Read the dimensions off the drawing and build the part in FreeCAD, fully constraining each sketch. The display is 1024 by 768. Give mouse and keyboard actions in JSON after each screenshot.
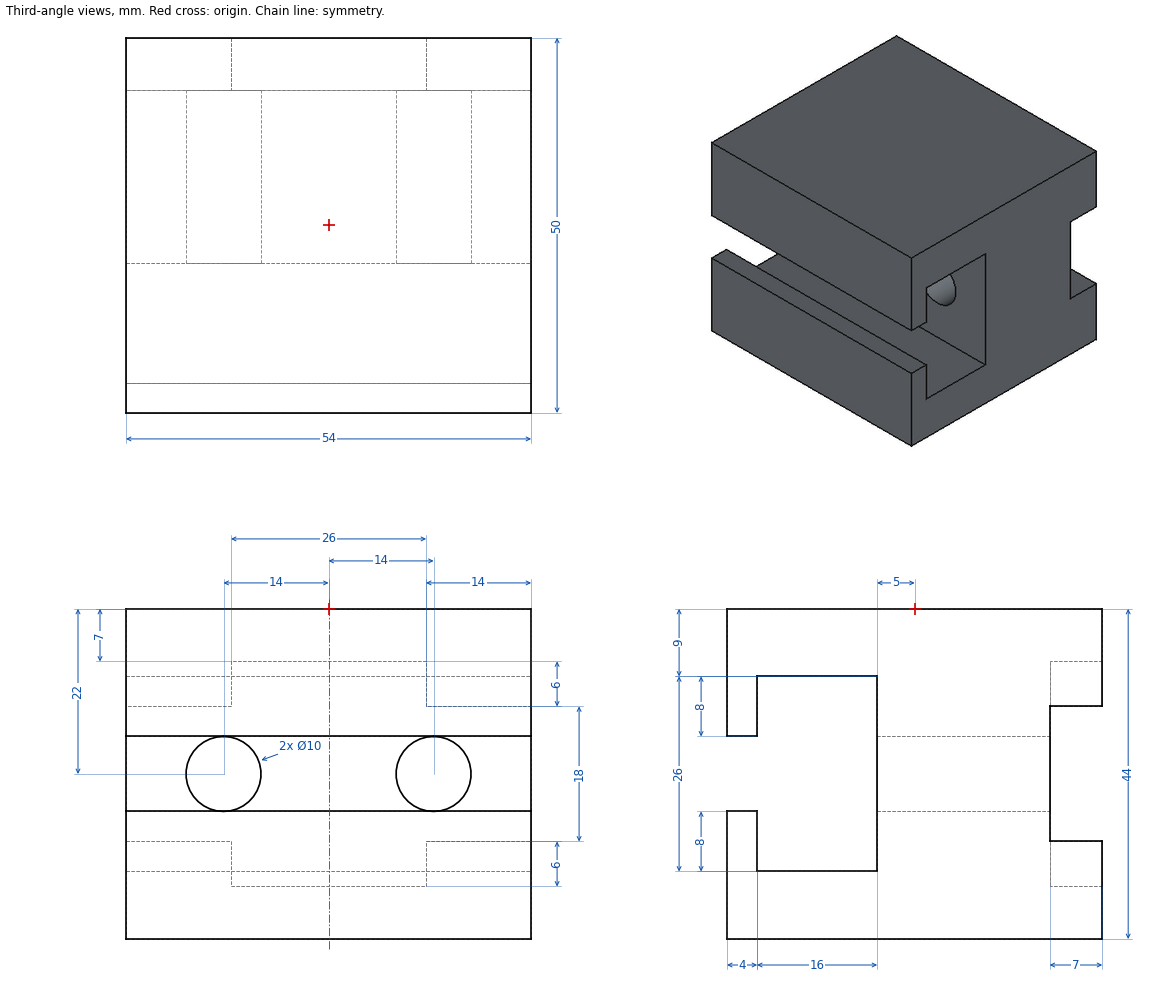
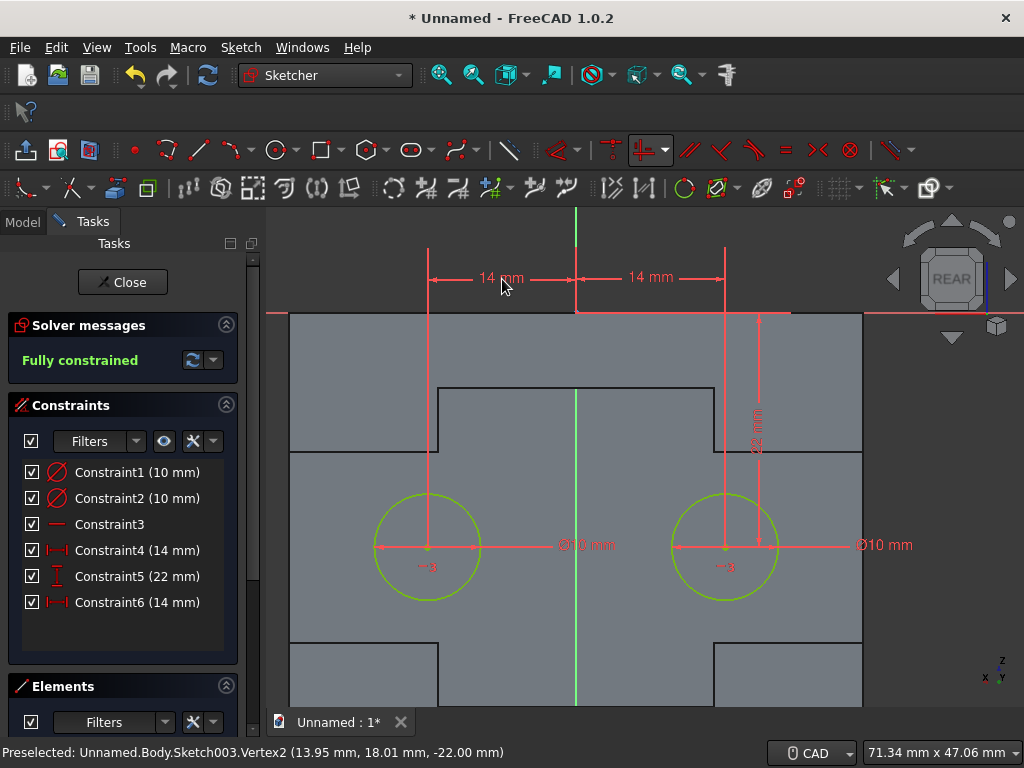
{"action": "left_click", "coordinate": [123, 282]}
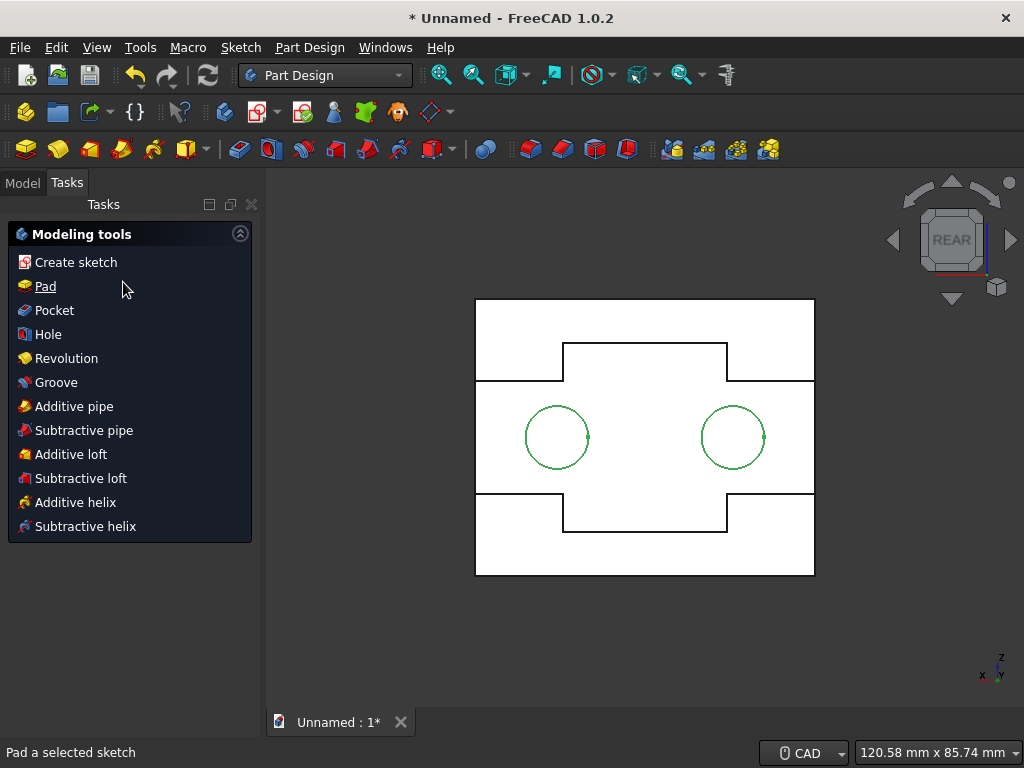
{"action": "left_click", "coordinate": [240, 150]}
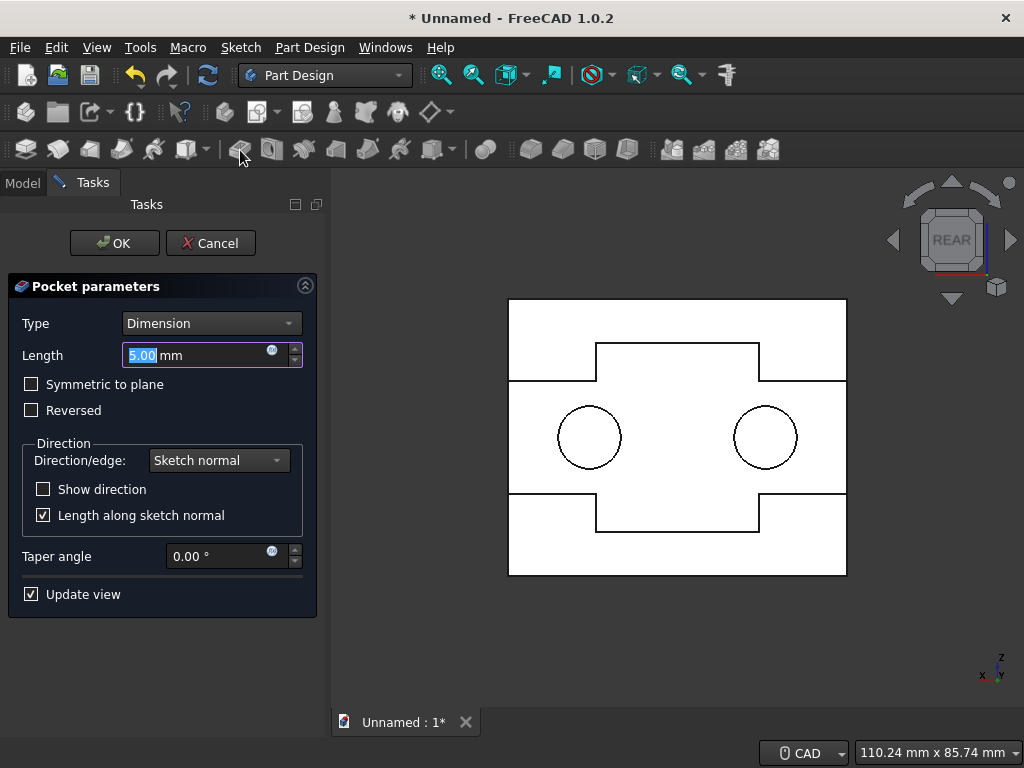
{"action": "left_click", "coordinate": [212, 324]}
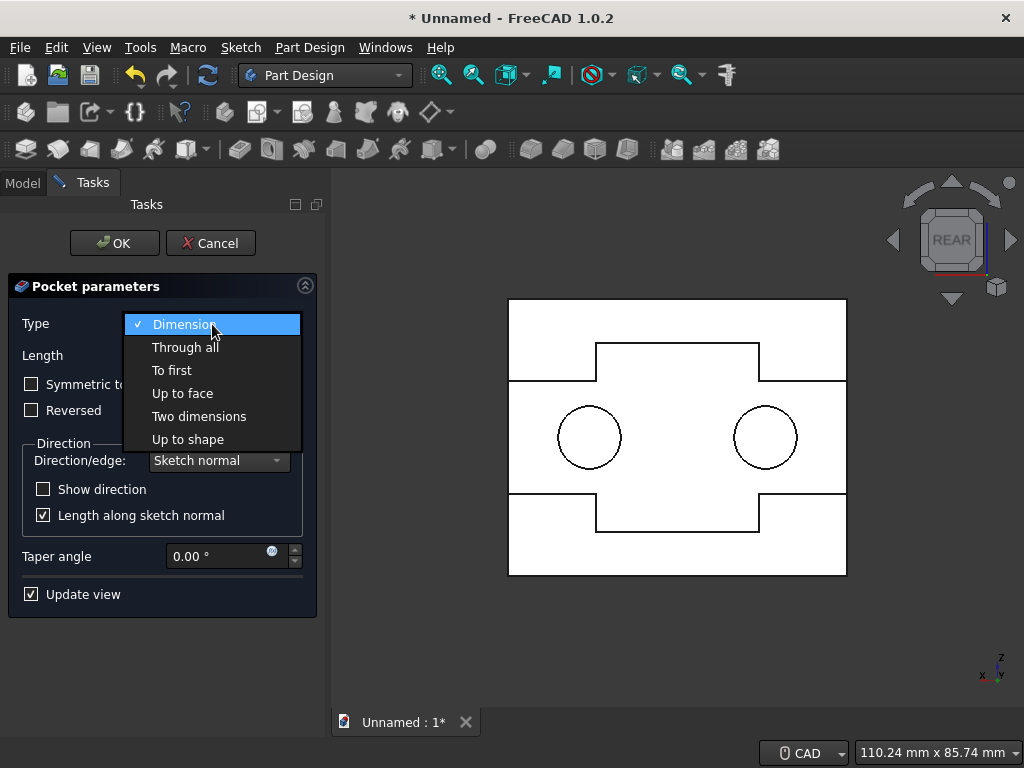
{"action": "left_click", "coordinate": [212, 348]}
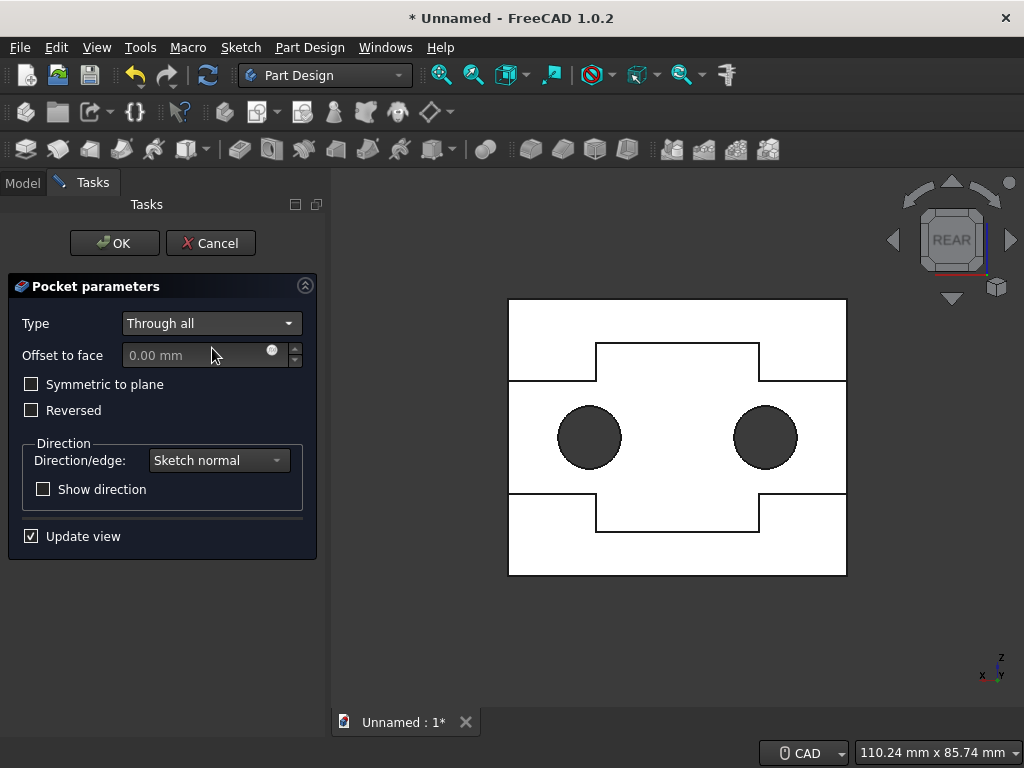
{"action": "left_click", "coordinate": [115, 243]}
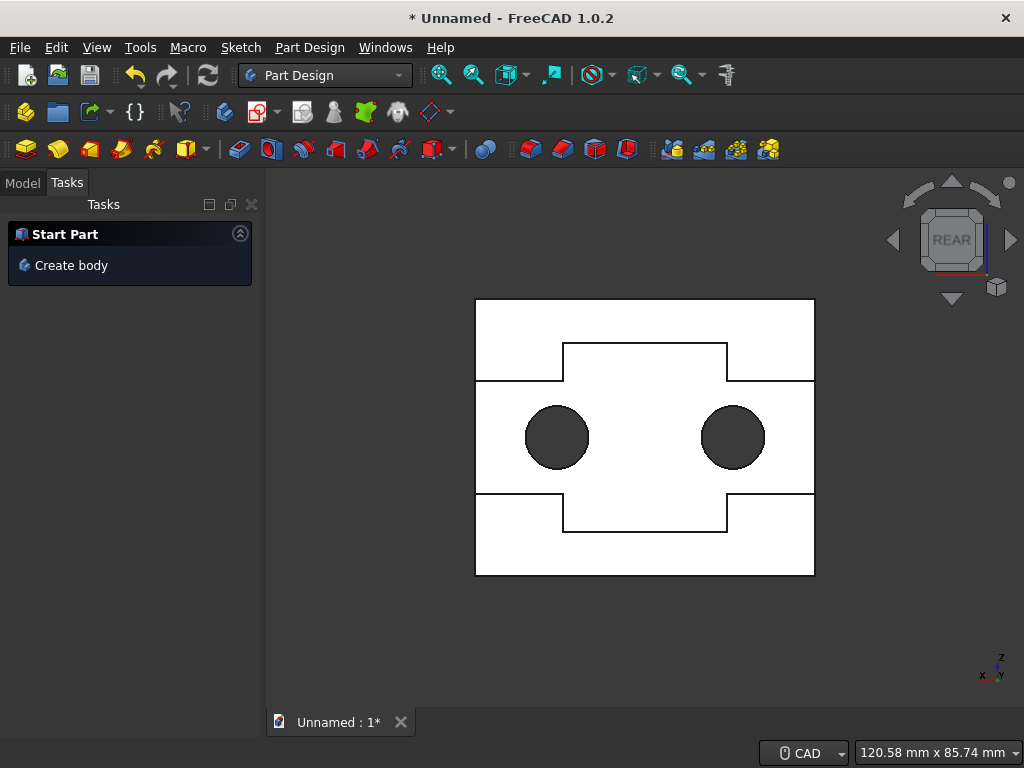
{"action": "key", "text": "0"}